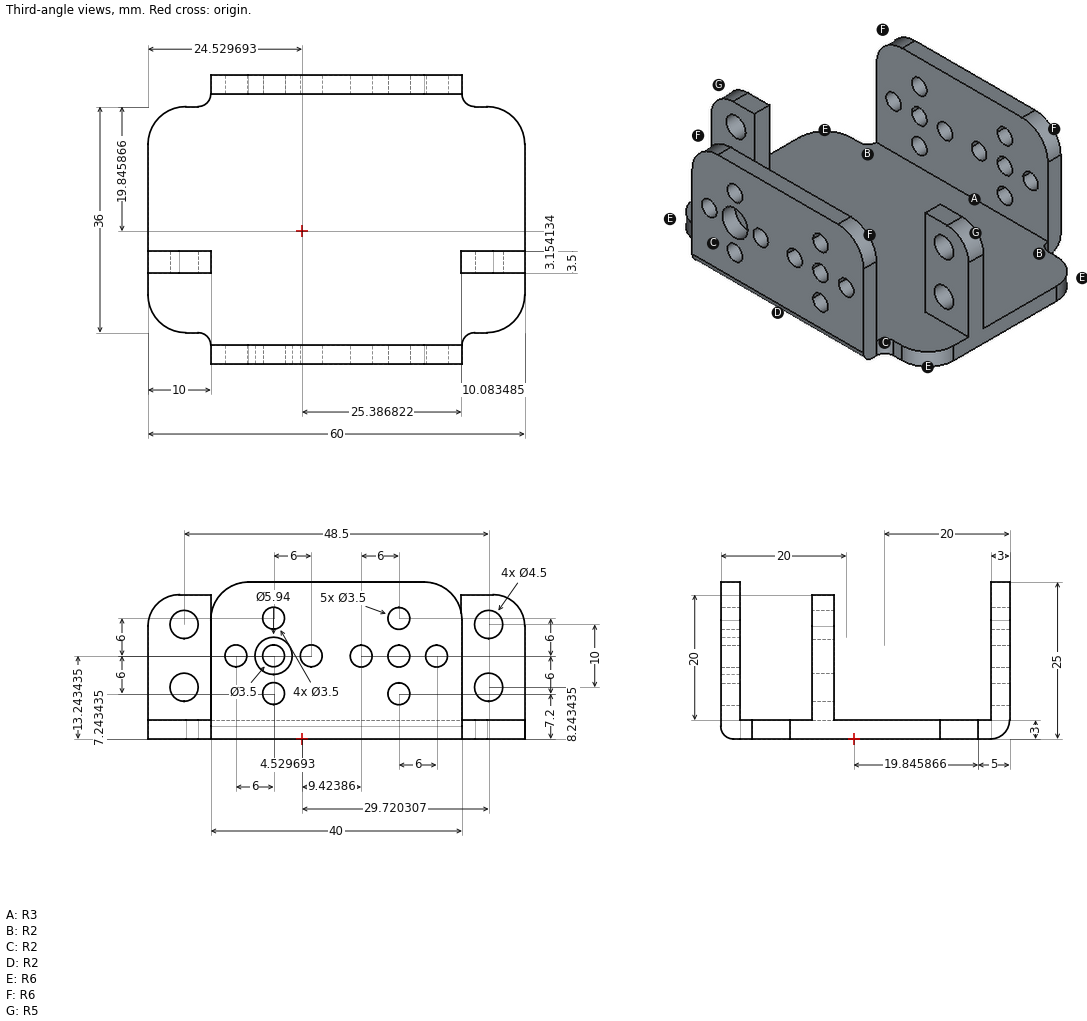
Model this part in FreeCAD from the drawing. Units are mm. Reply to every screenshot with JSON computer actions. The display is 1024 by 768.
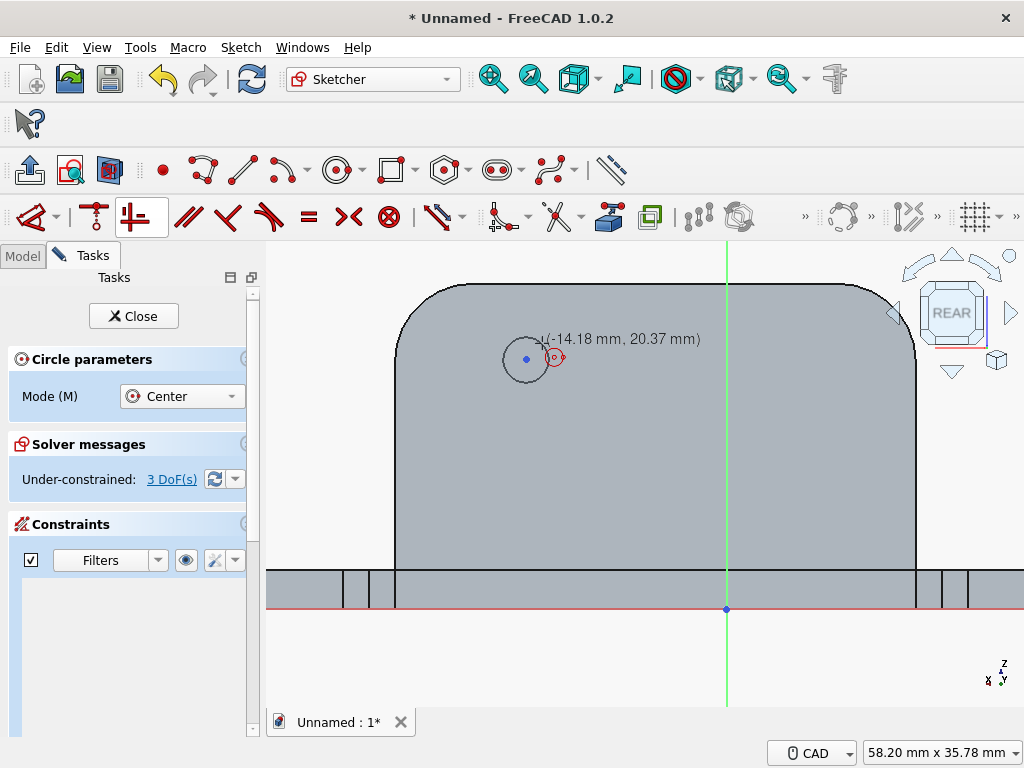
{"action": "left_click", "coordinate": [604, 437]}
{"action": "left_click", "coordinate": [620, 421]}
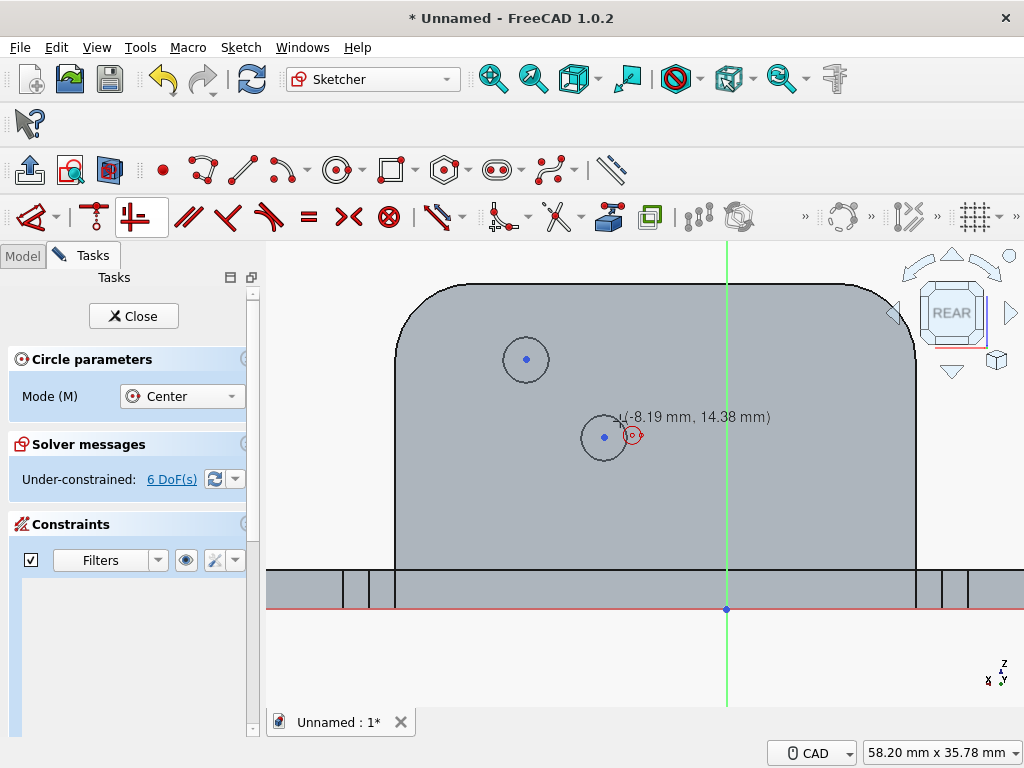
{"action": "left_click", "coordinate": [526, 516]}
{"action": "left_click", "coordinate": [542, 499]}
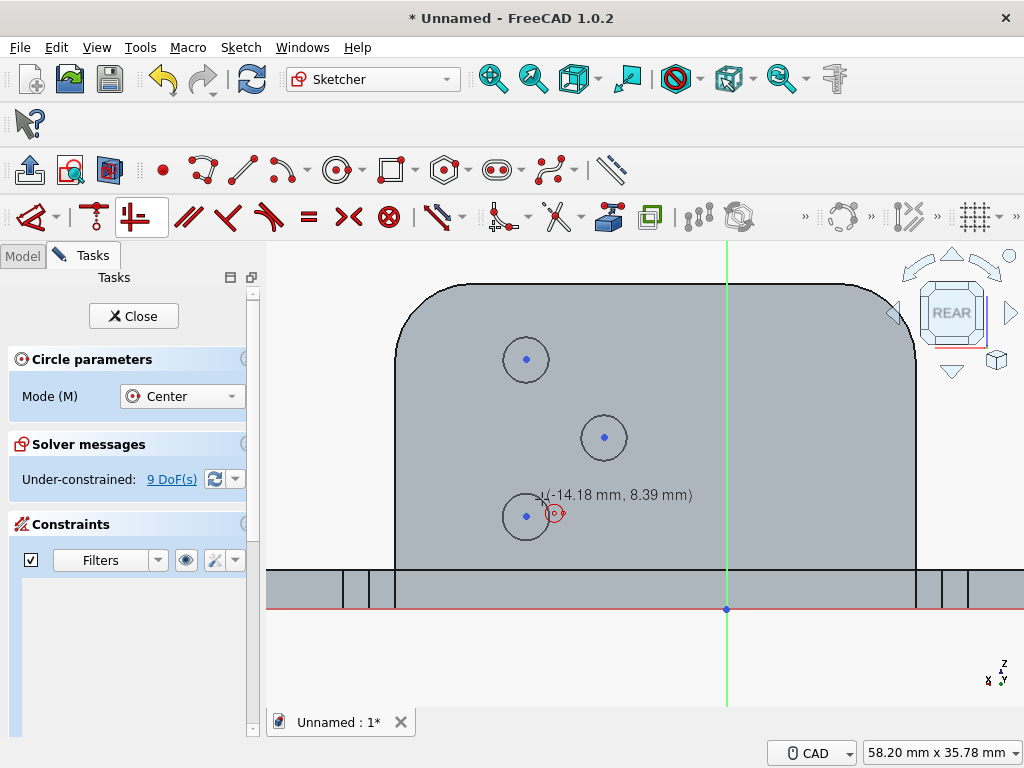
{"action": "left_click", "coordinate": [448, 437]}
{"action": "left_click", "coordinate": [464, 421]}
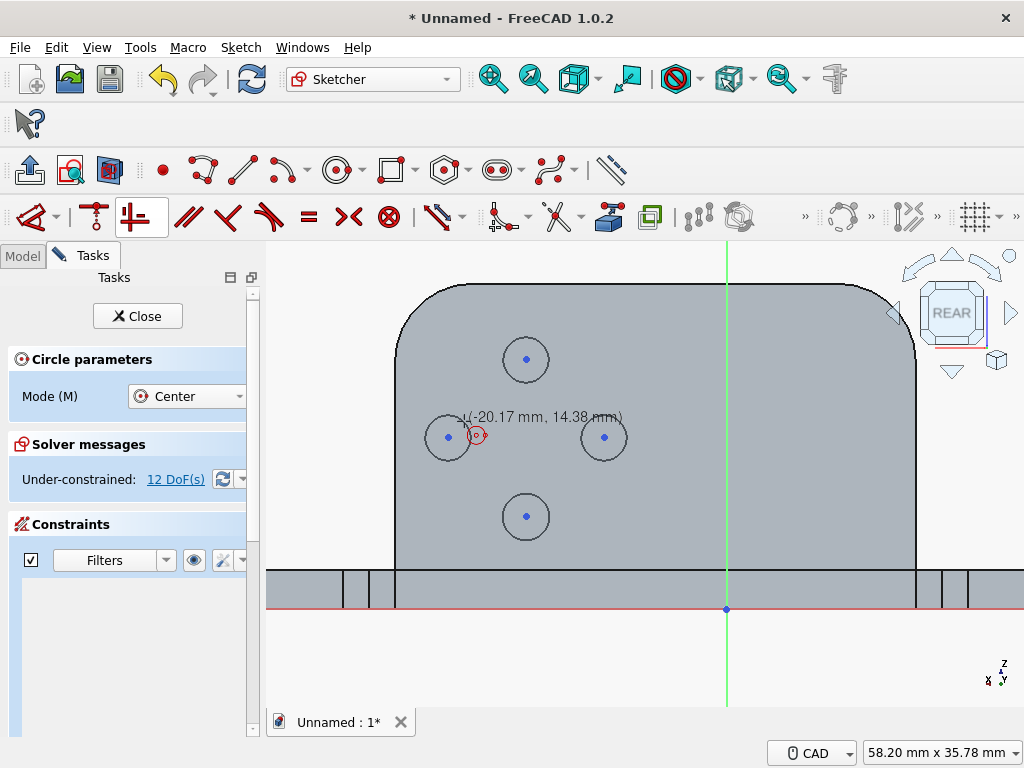
{"action": "left_click", "coordinate": [526, 437]}
{"action": "left_click", "coordinate": [542, 421]}
{"action": "key", "text": "Escape"}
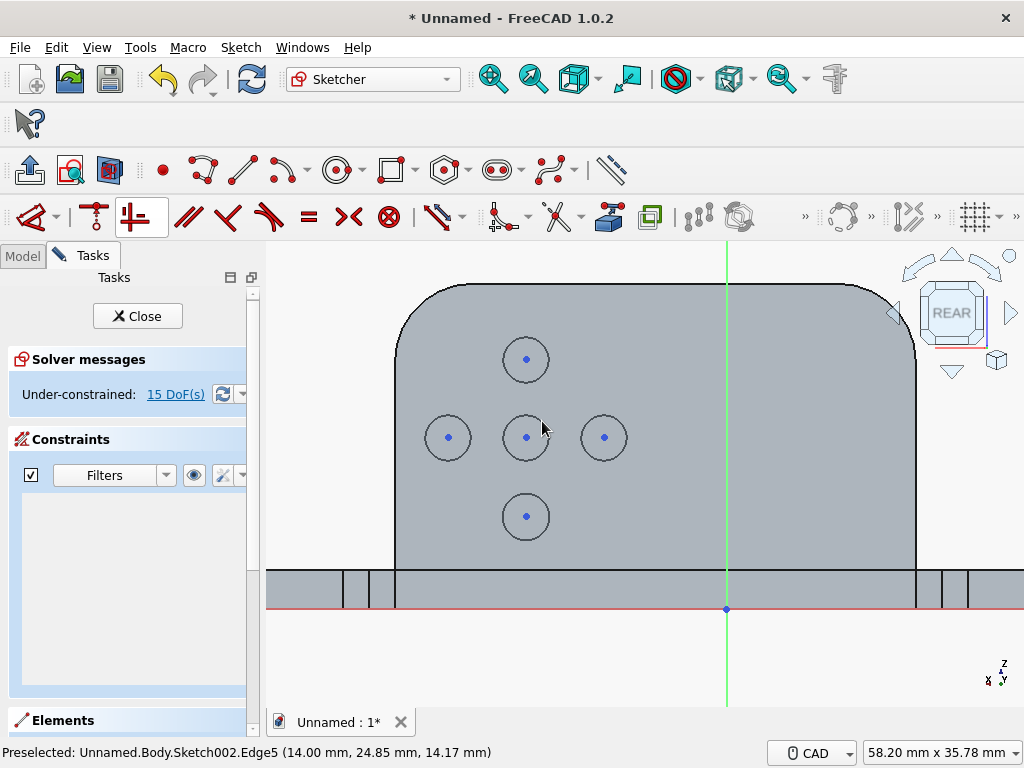
{"action": "left_click", "coordinate": [542, 344]}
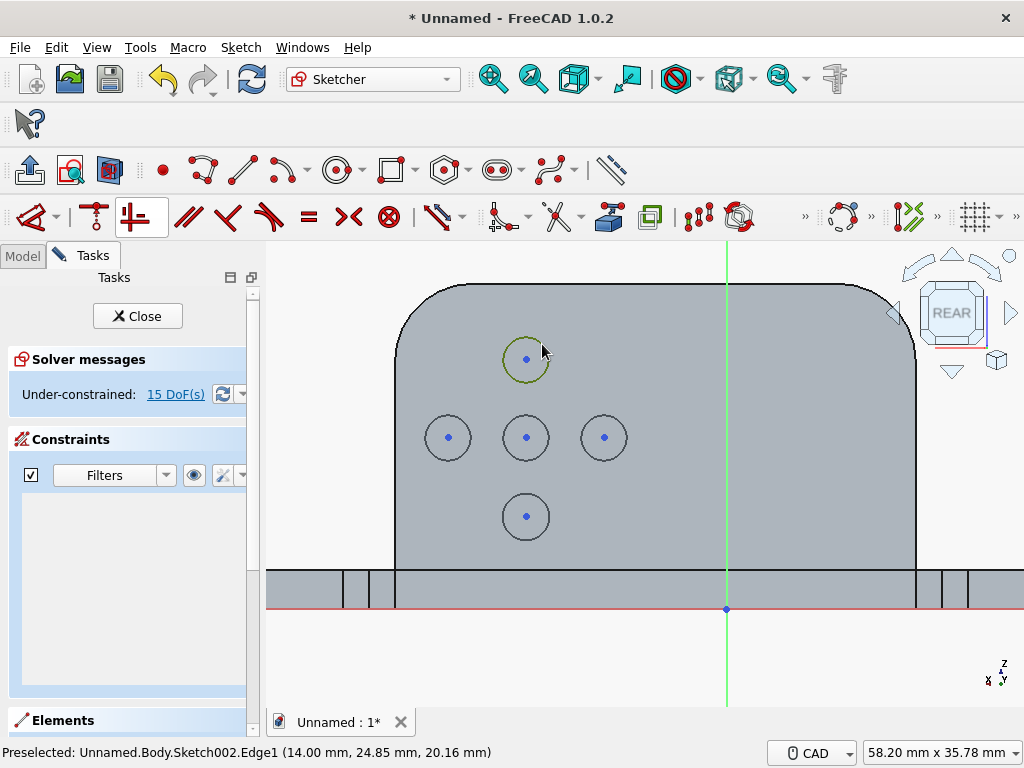
{"action": "left_click", "coordinate": [620, 422]}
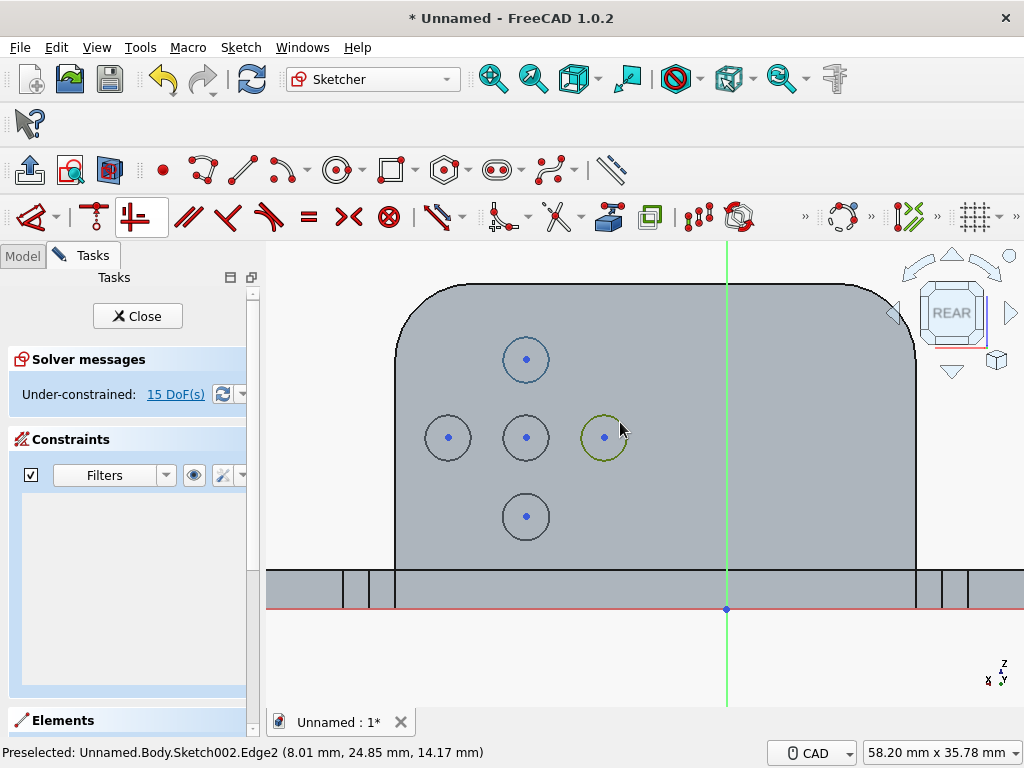
{"action": "left_click", "coordinate": [542, 500]}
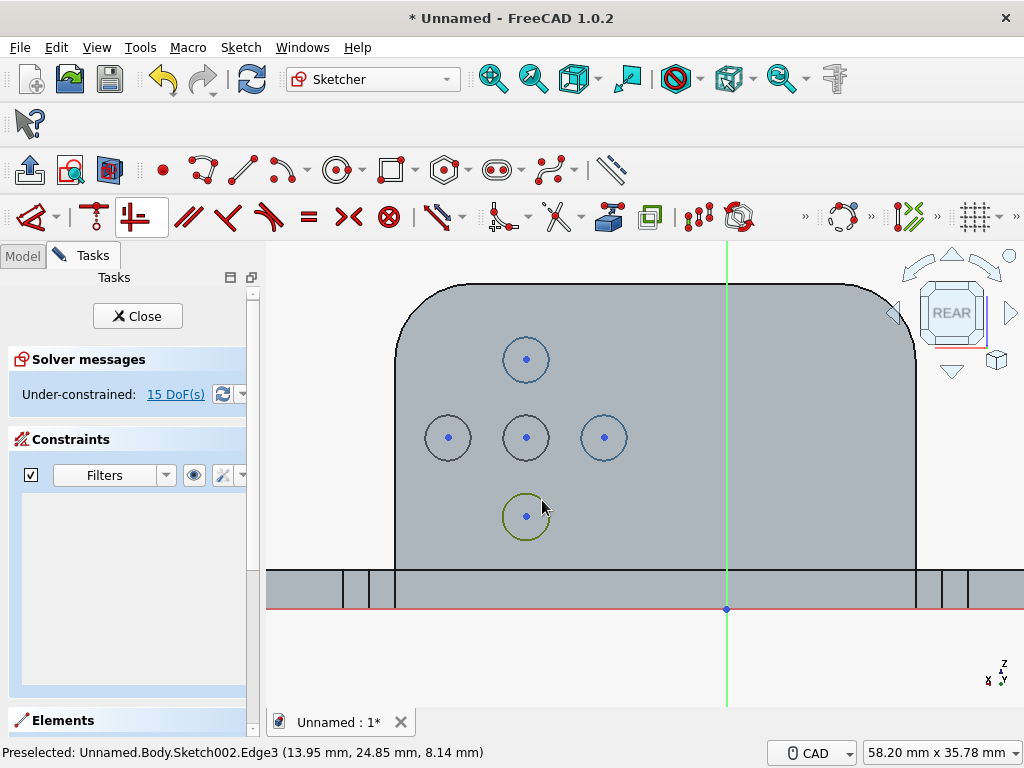
{"action": "left_click", "coordinate": [464, 422]}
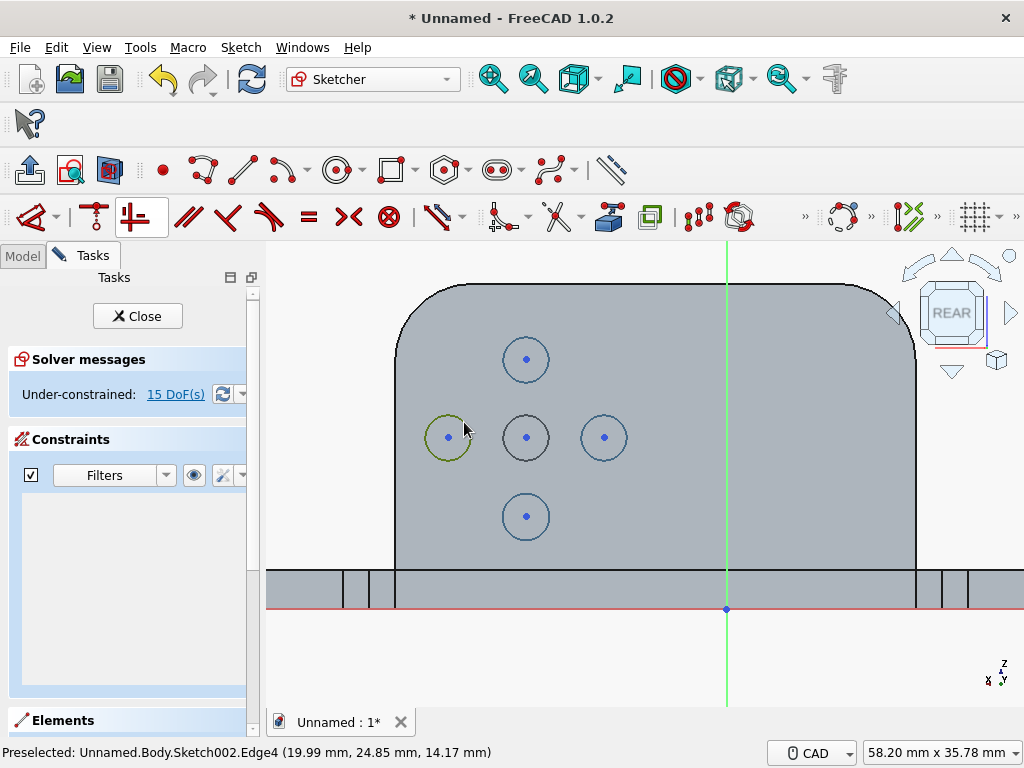
{"action": "left_click", "coordinate": [542, 422]}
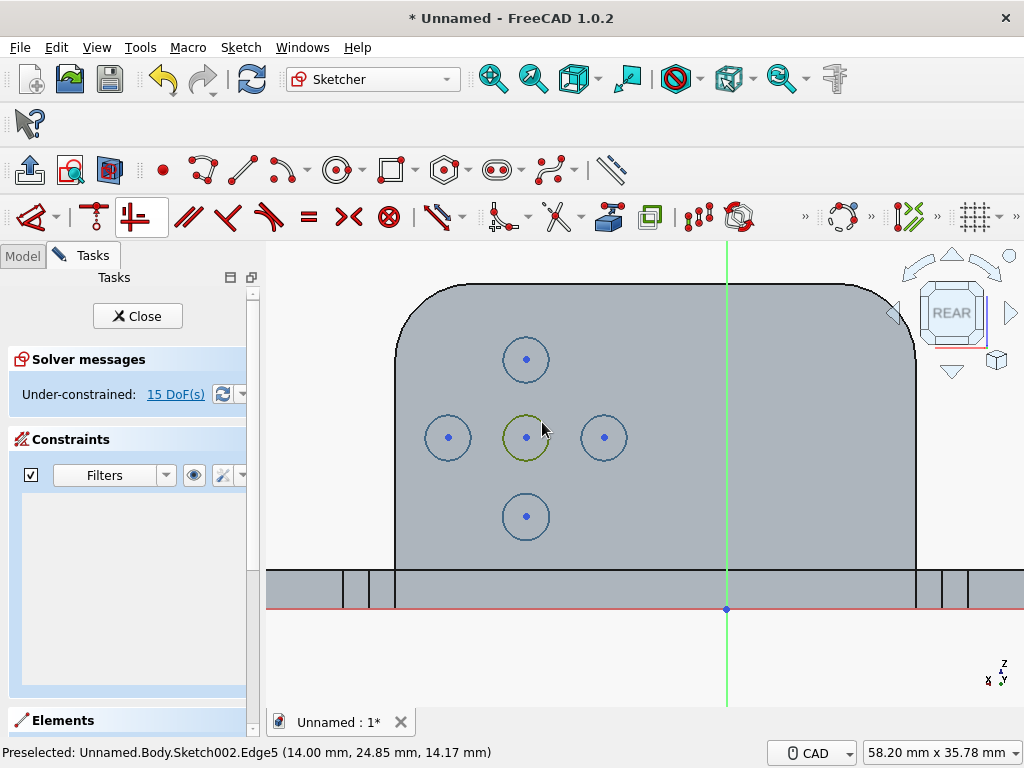
{"action": "left_click", "coordinate": [310, 218]}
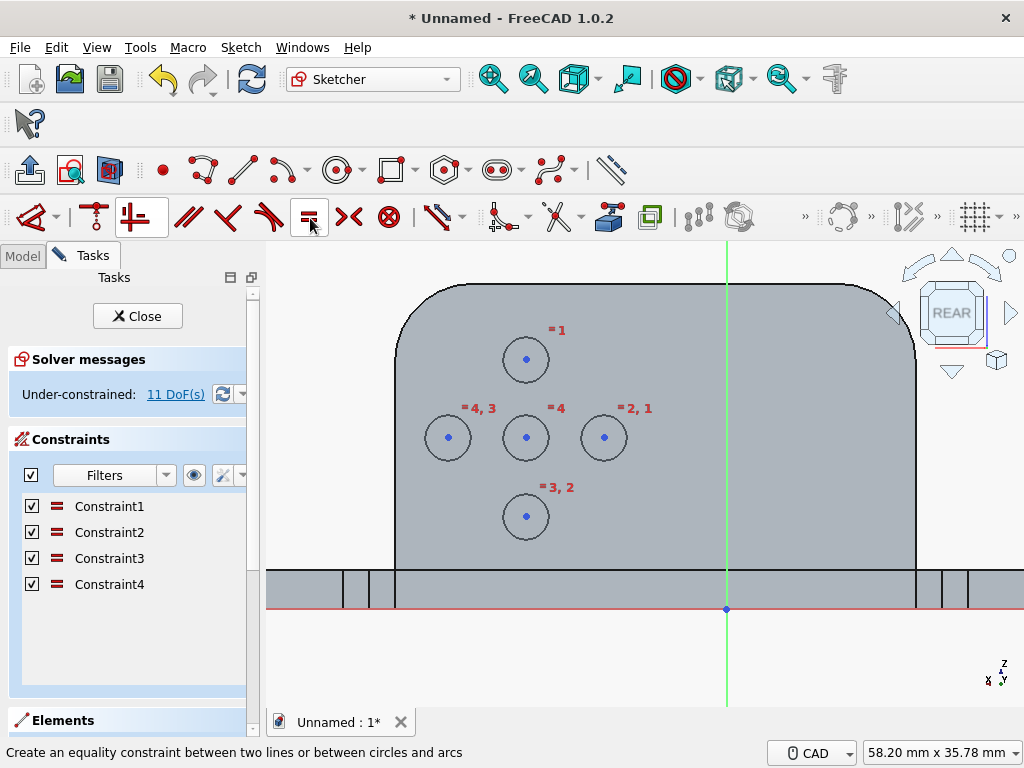
{"action": "left_click", "coordinate": [526, 360]}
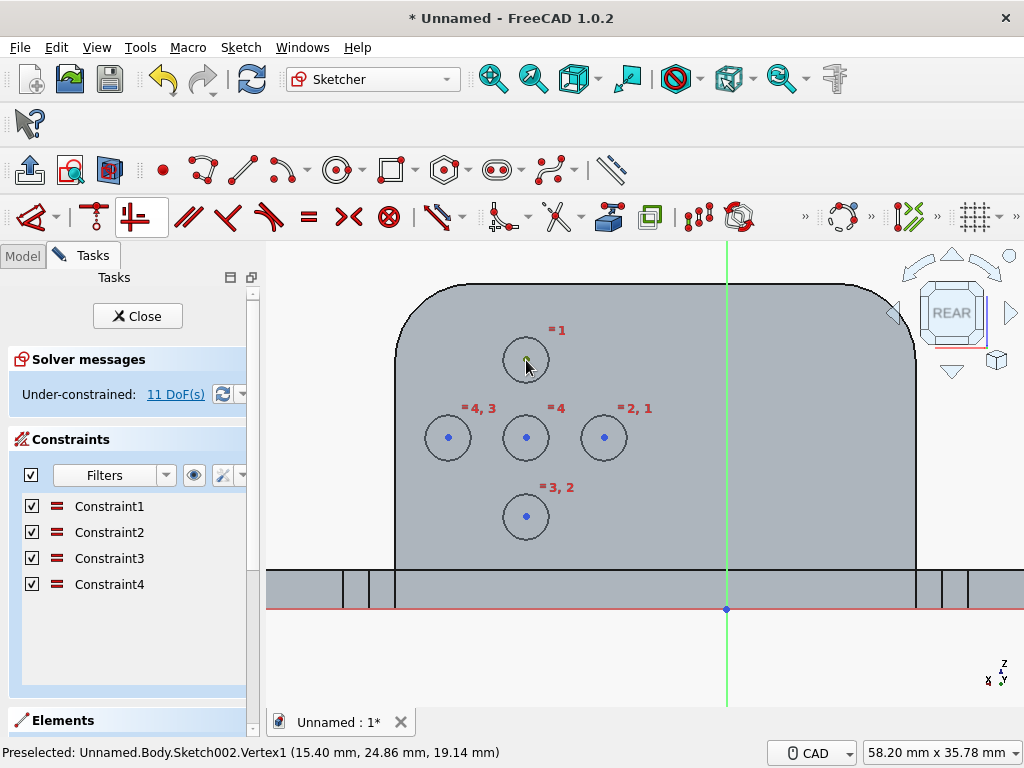
{"action": "left_click", "coordinate": [526, 517]}